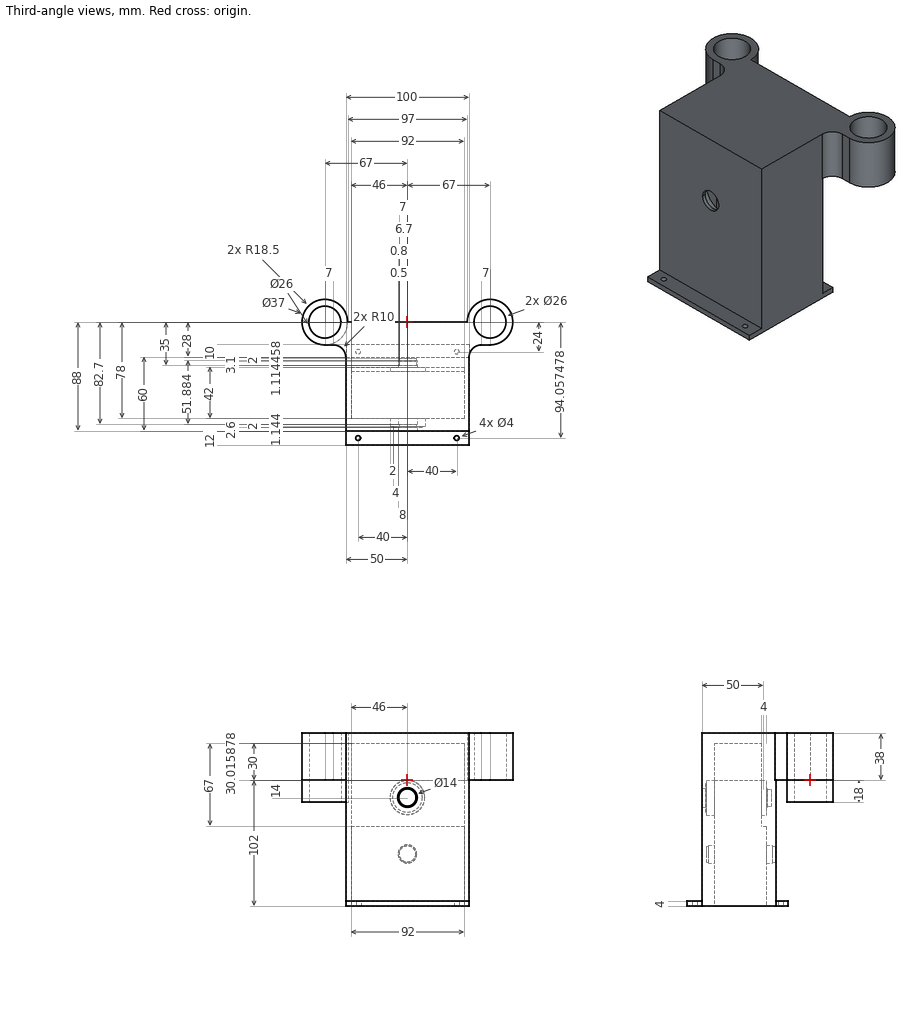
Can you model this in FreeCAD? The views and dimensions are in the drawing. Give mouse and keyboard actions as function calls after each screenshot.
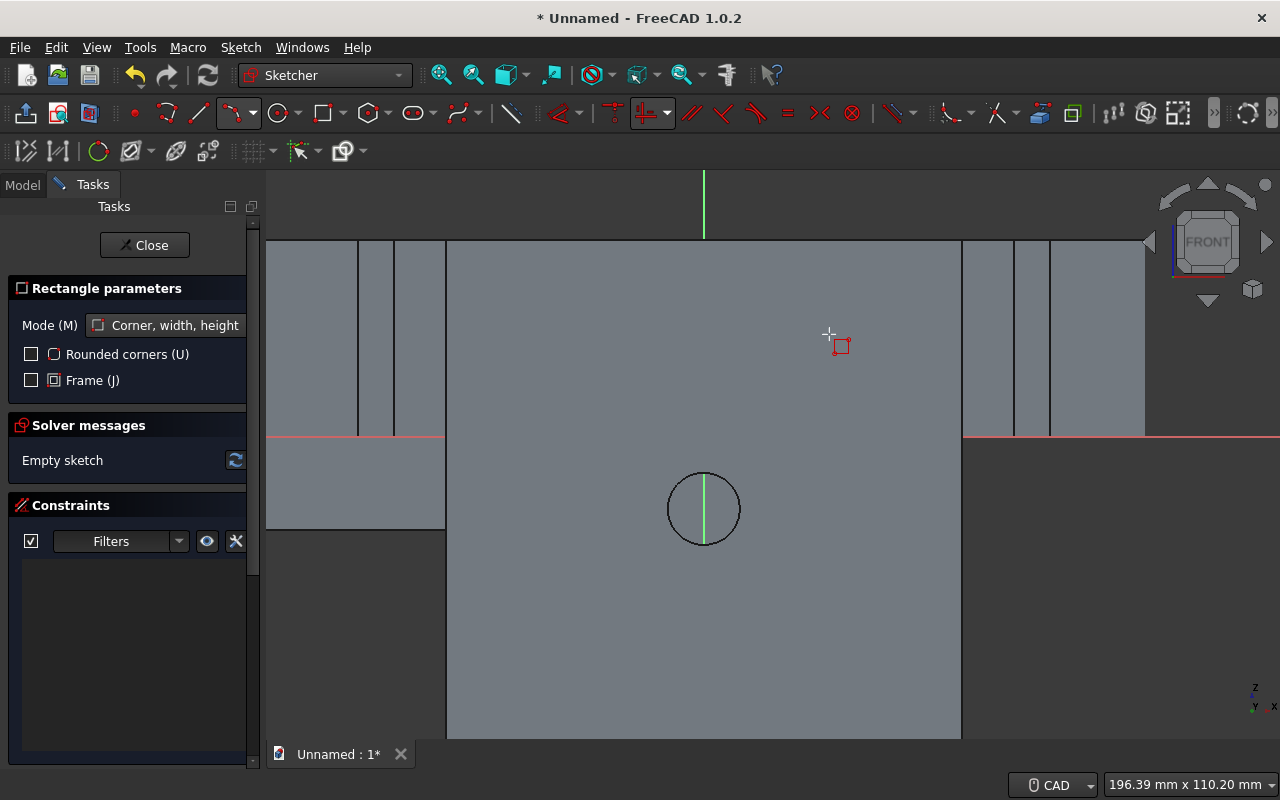
click(466, 282)
click(941, 628)
key(Escape)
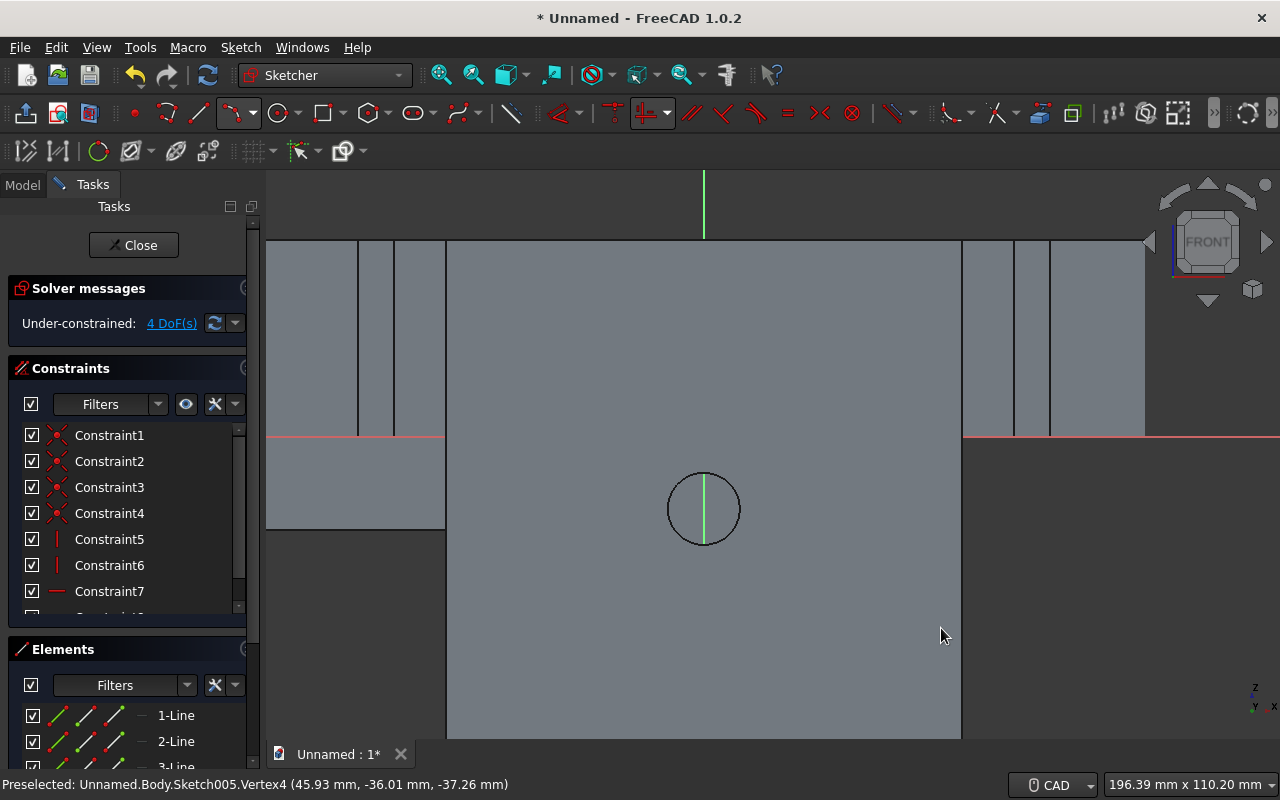
key(d)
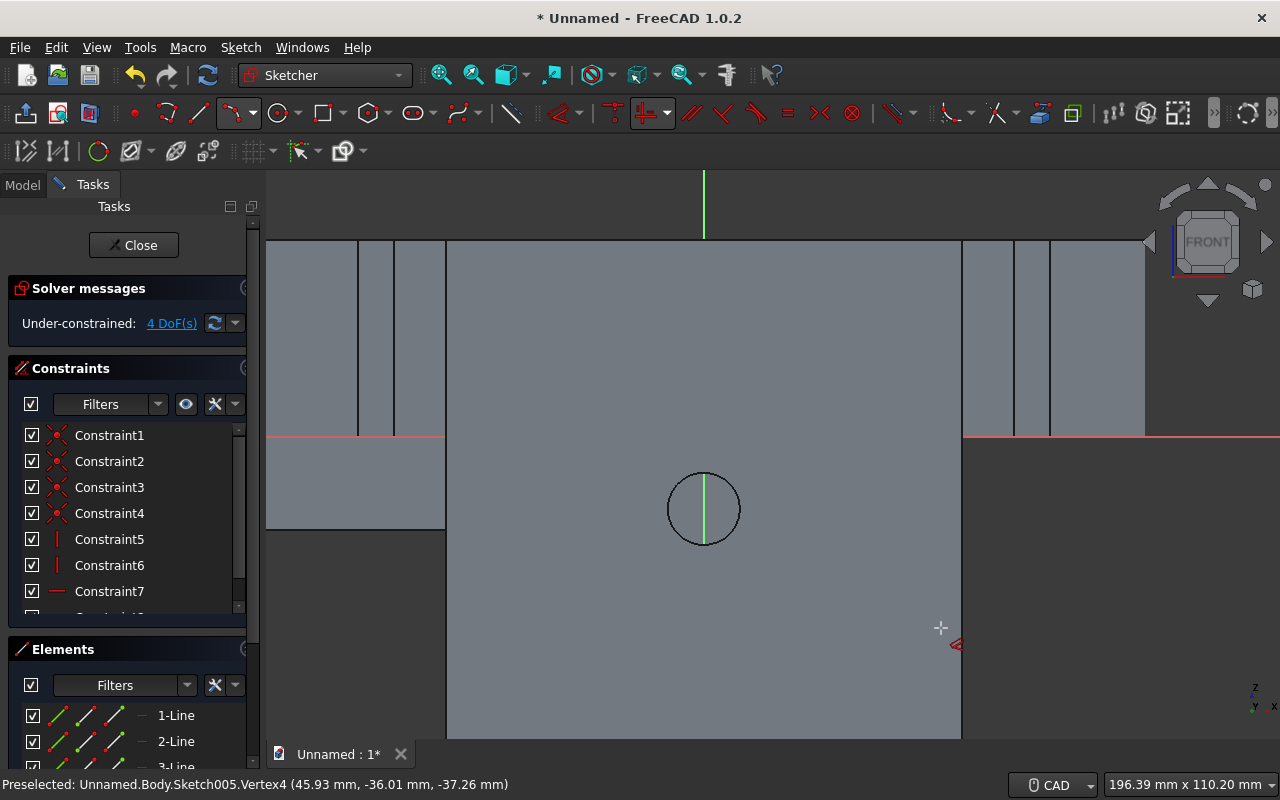
click(466, 387)
click(432, 456)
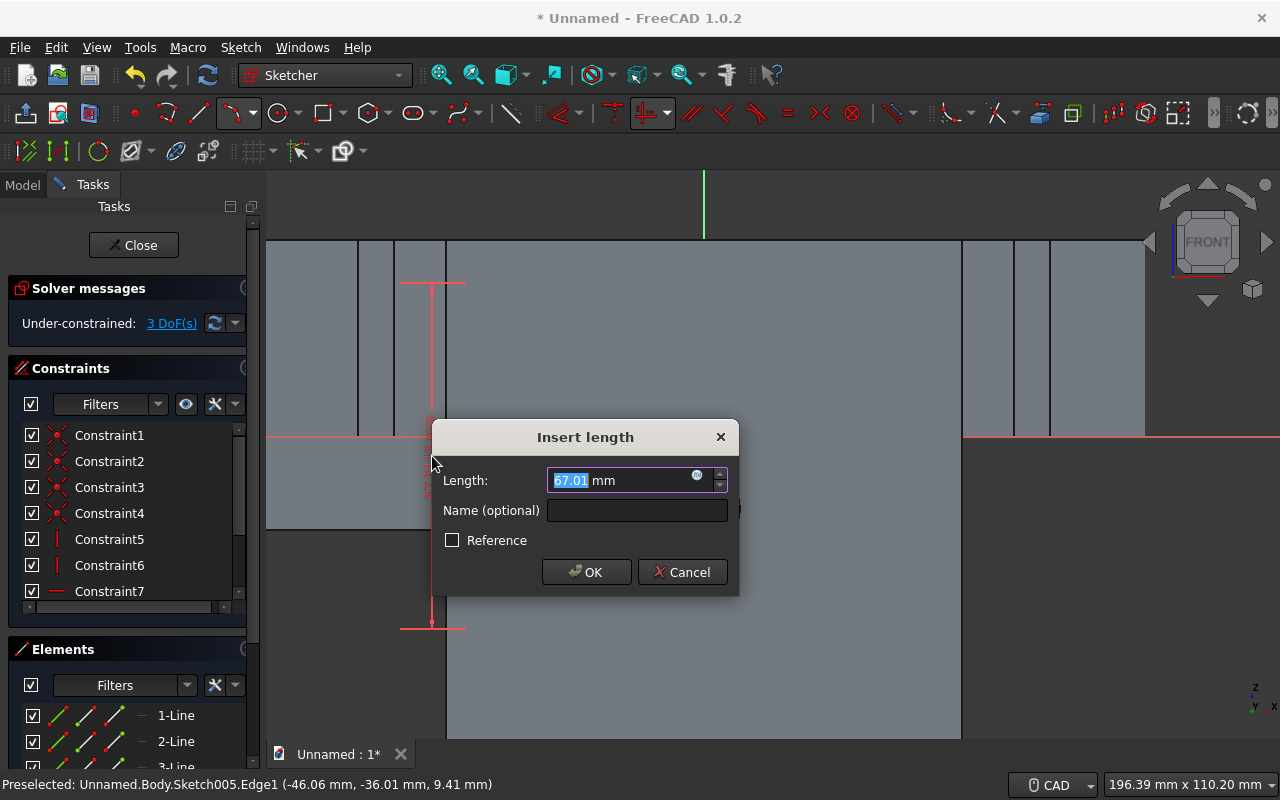
text(67)
key(Return)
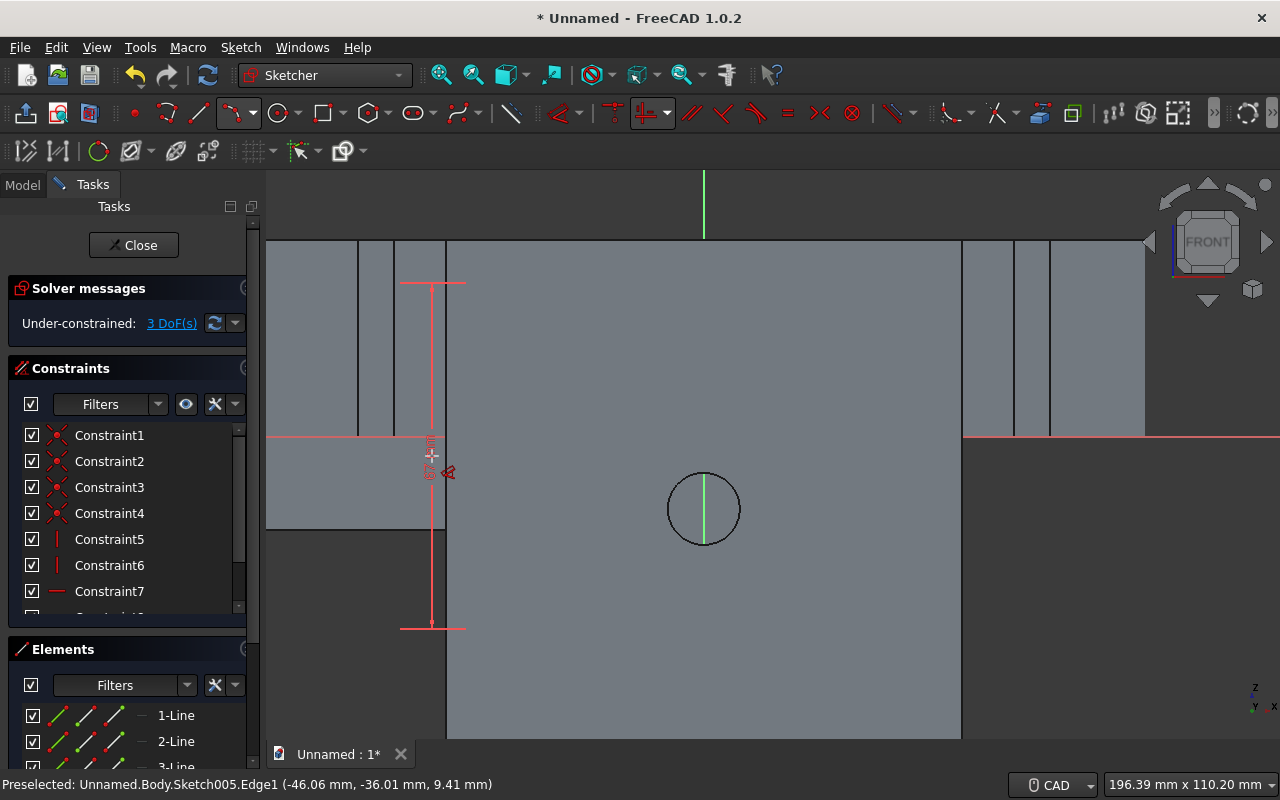
click(608, 629)
click(594, 663)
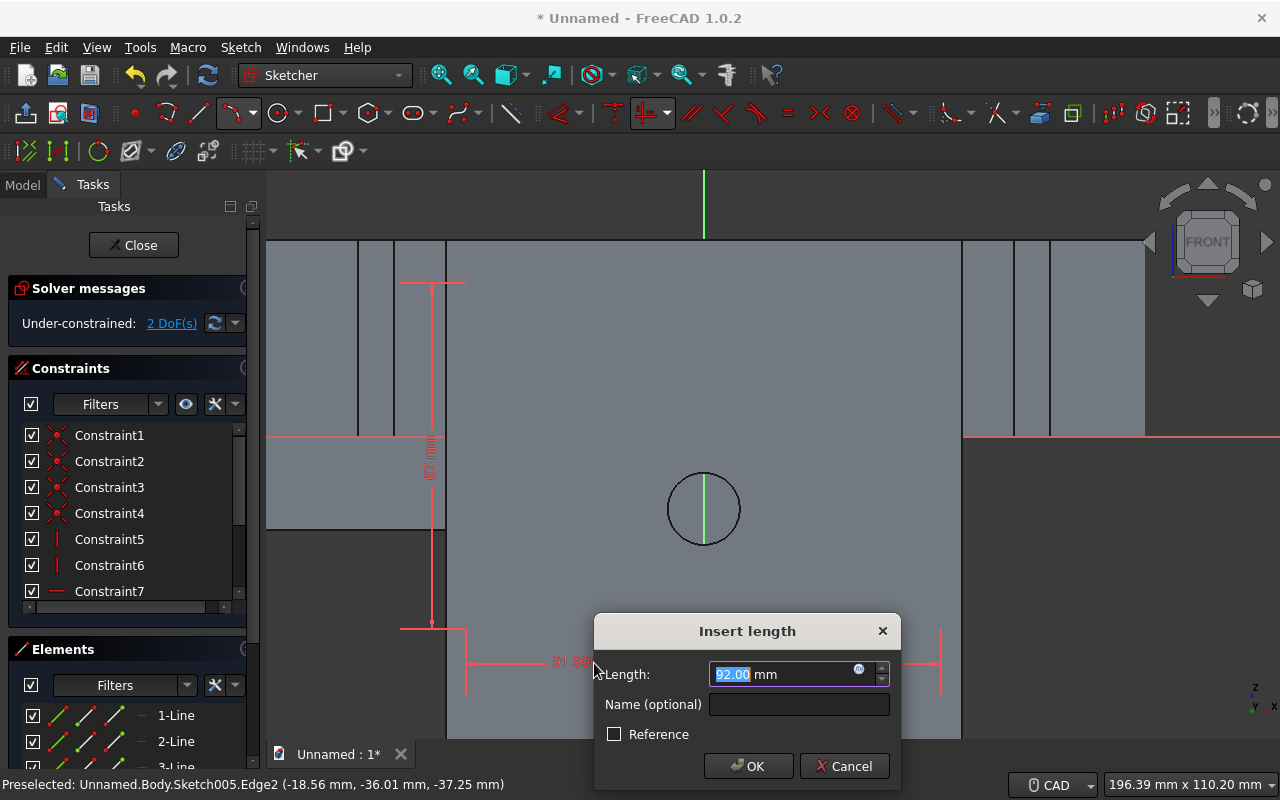
text(92)
key(Return)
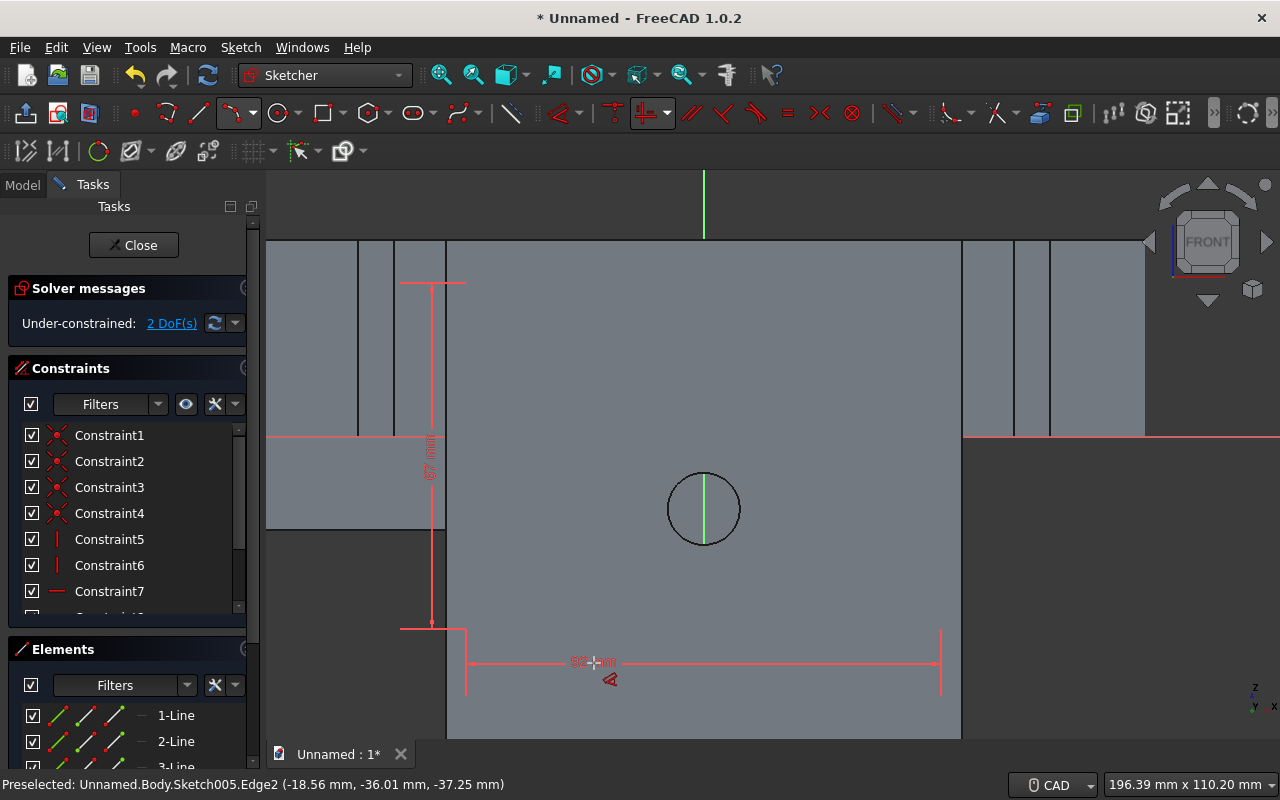
click(466, 283)
click(585, 249)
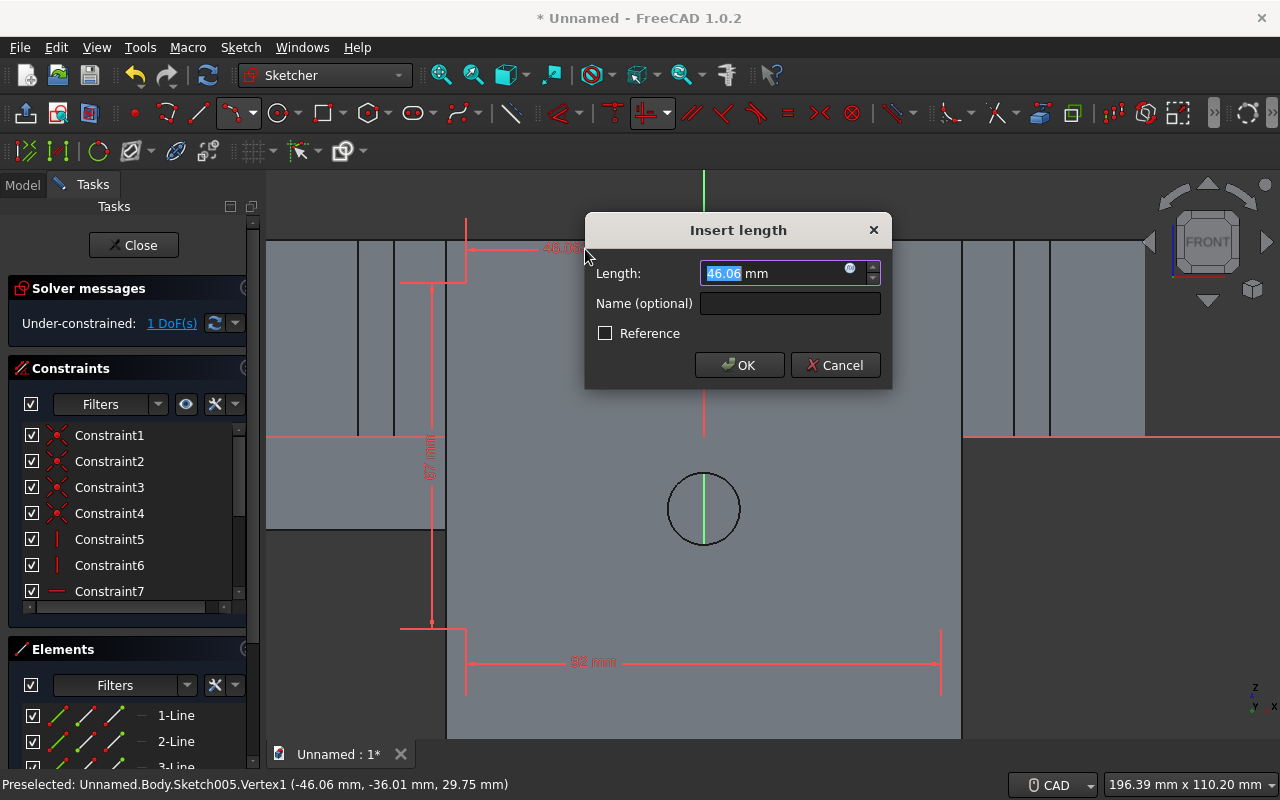
text(46)
key(Return)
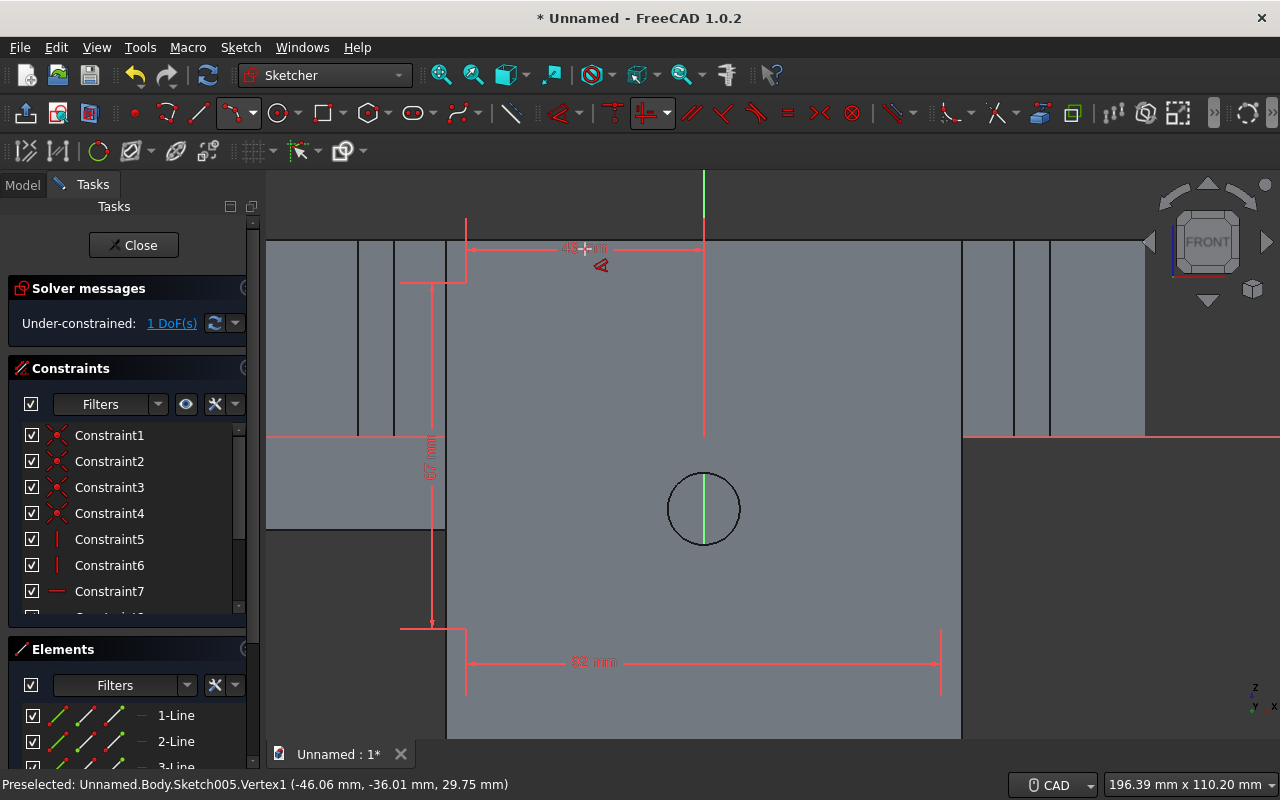
click(466, 283)
click(432, 360)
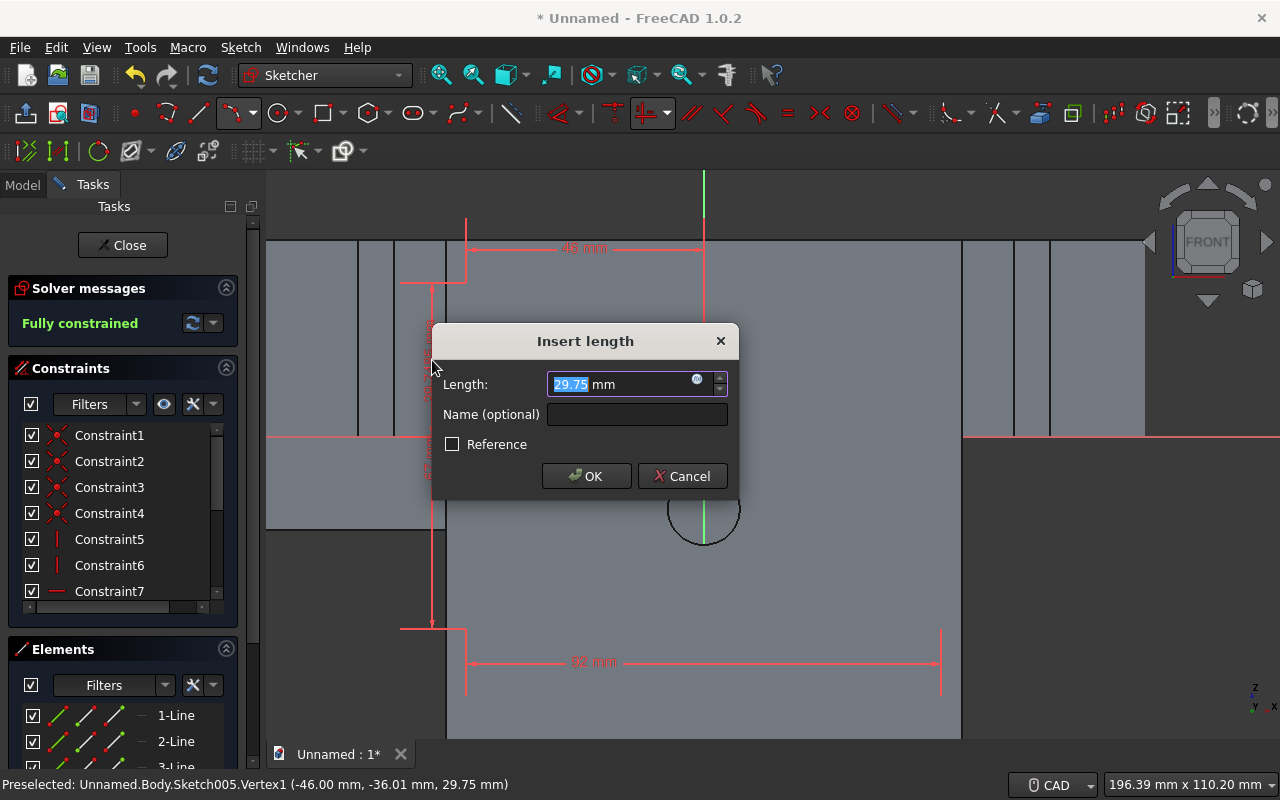
text(30.015878)
key(Return)
key(Escape)